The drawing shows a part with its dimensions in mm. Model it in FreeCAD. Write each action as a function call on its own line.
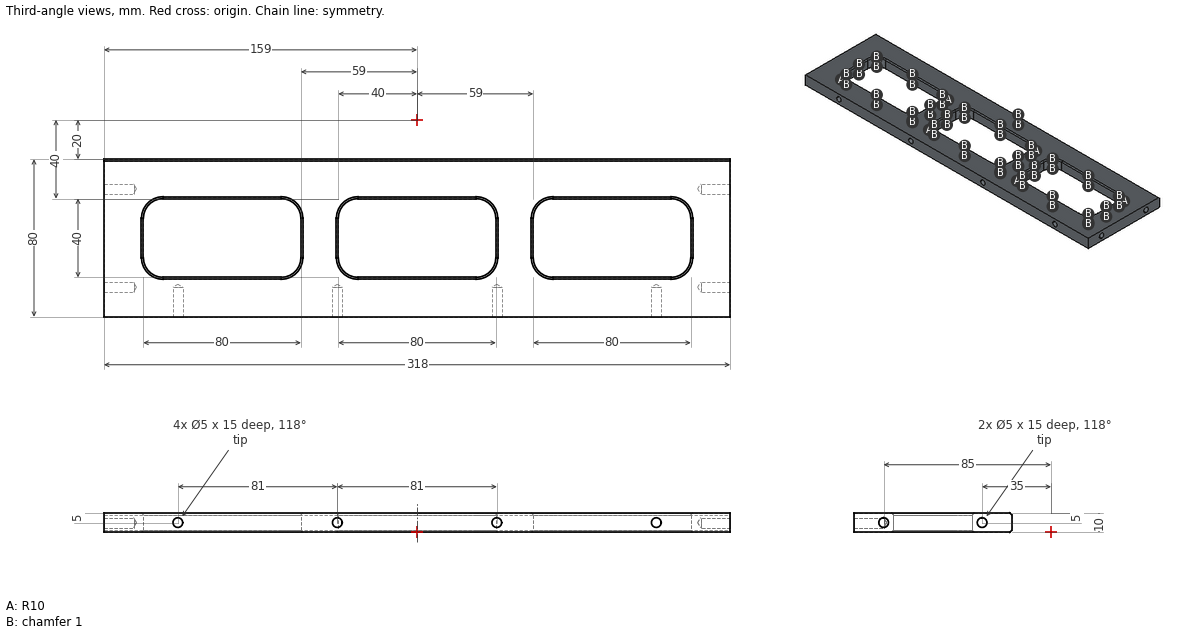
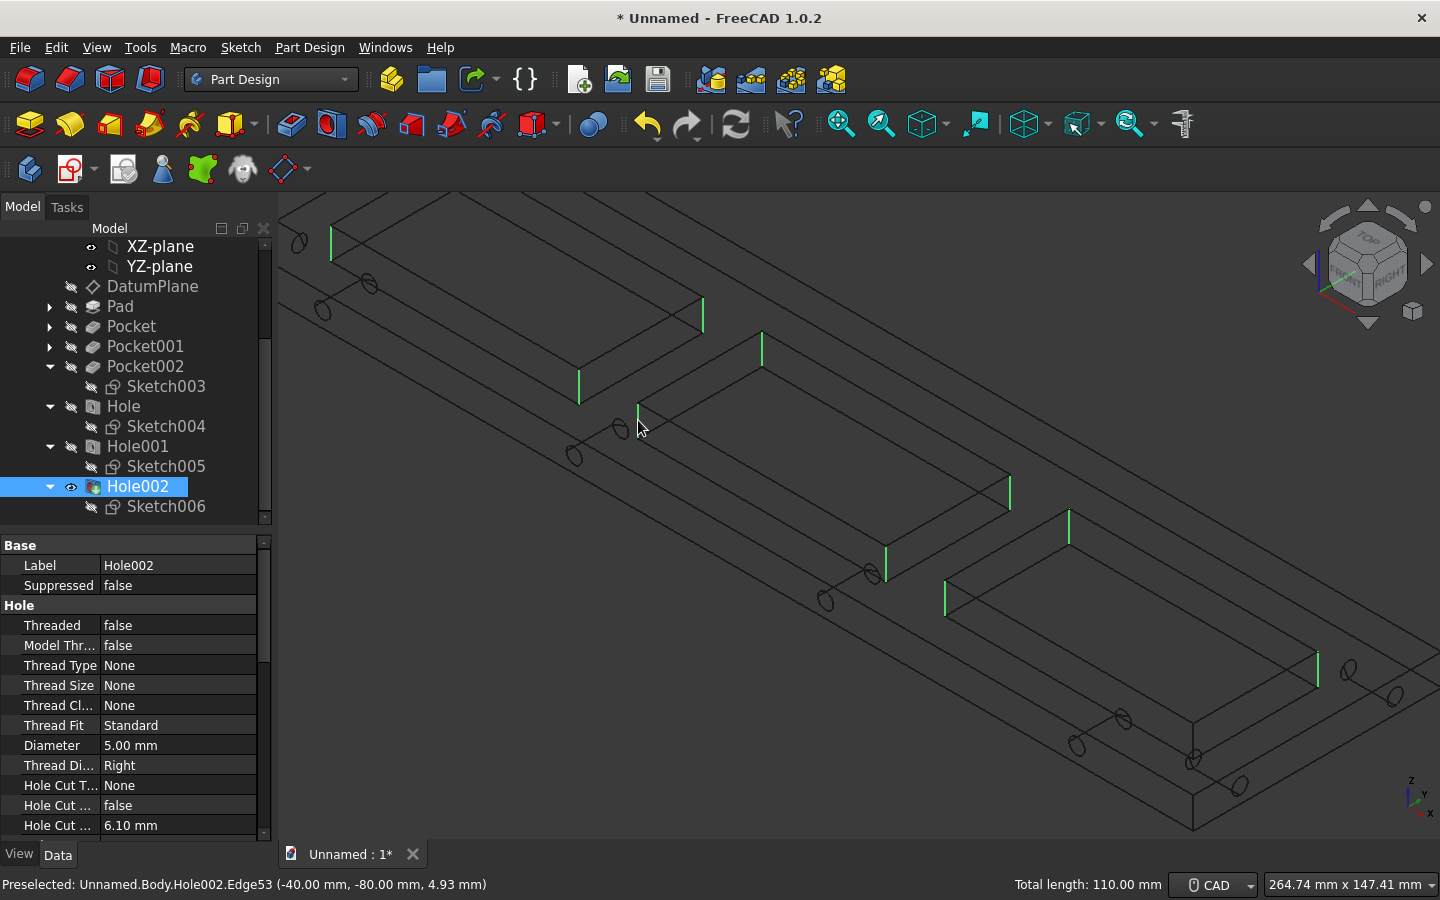
click(1193, 740, ctrl)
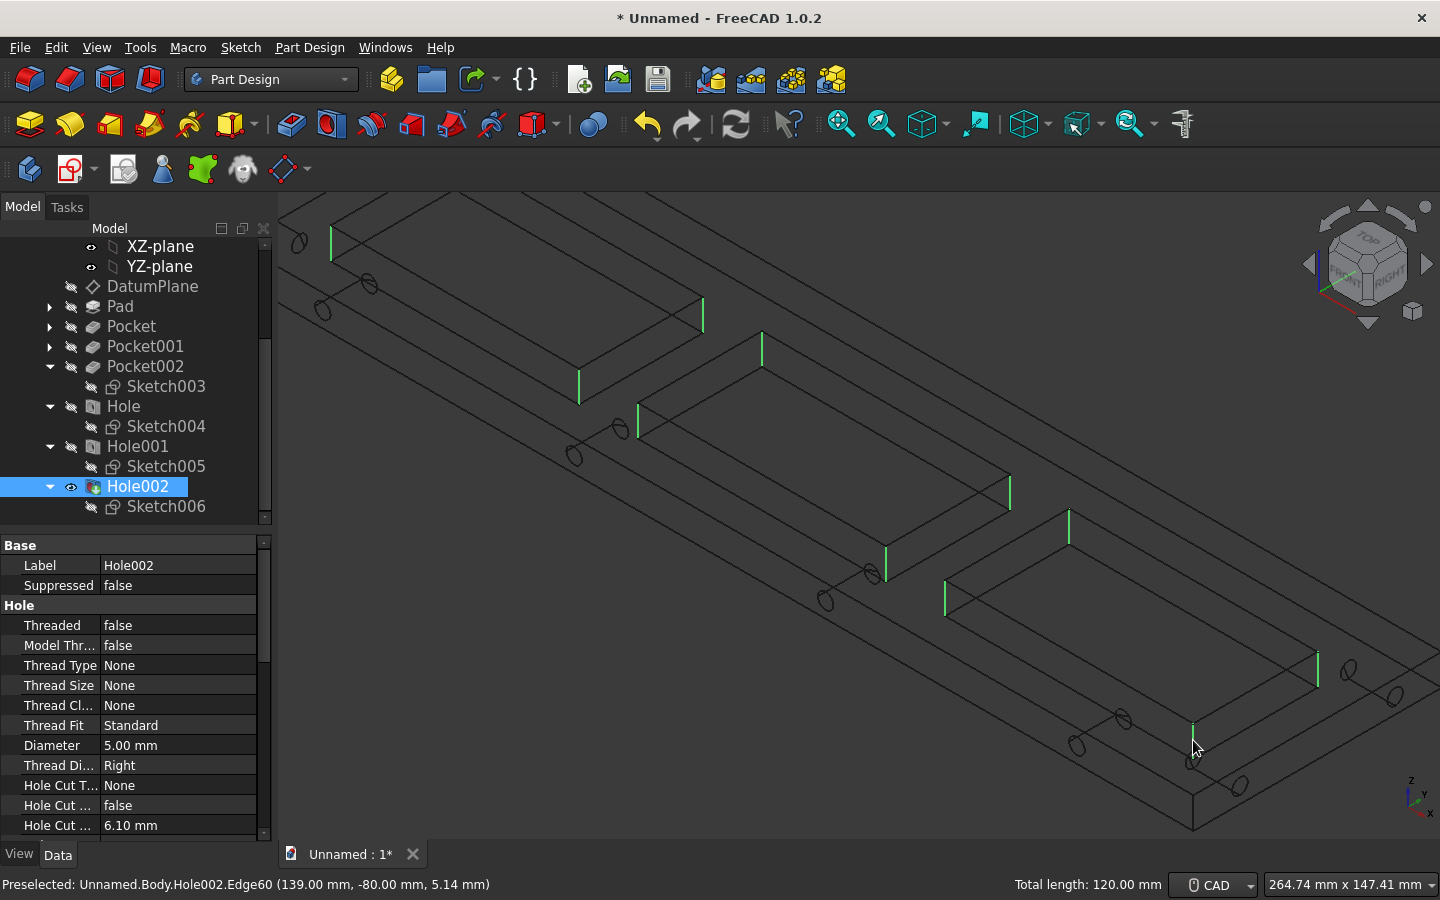
key(v)
key(1)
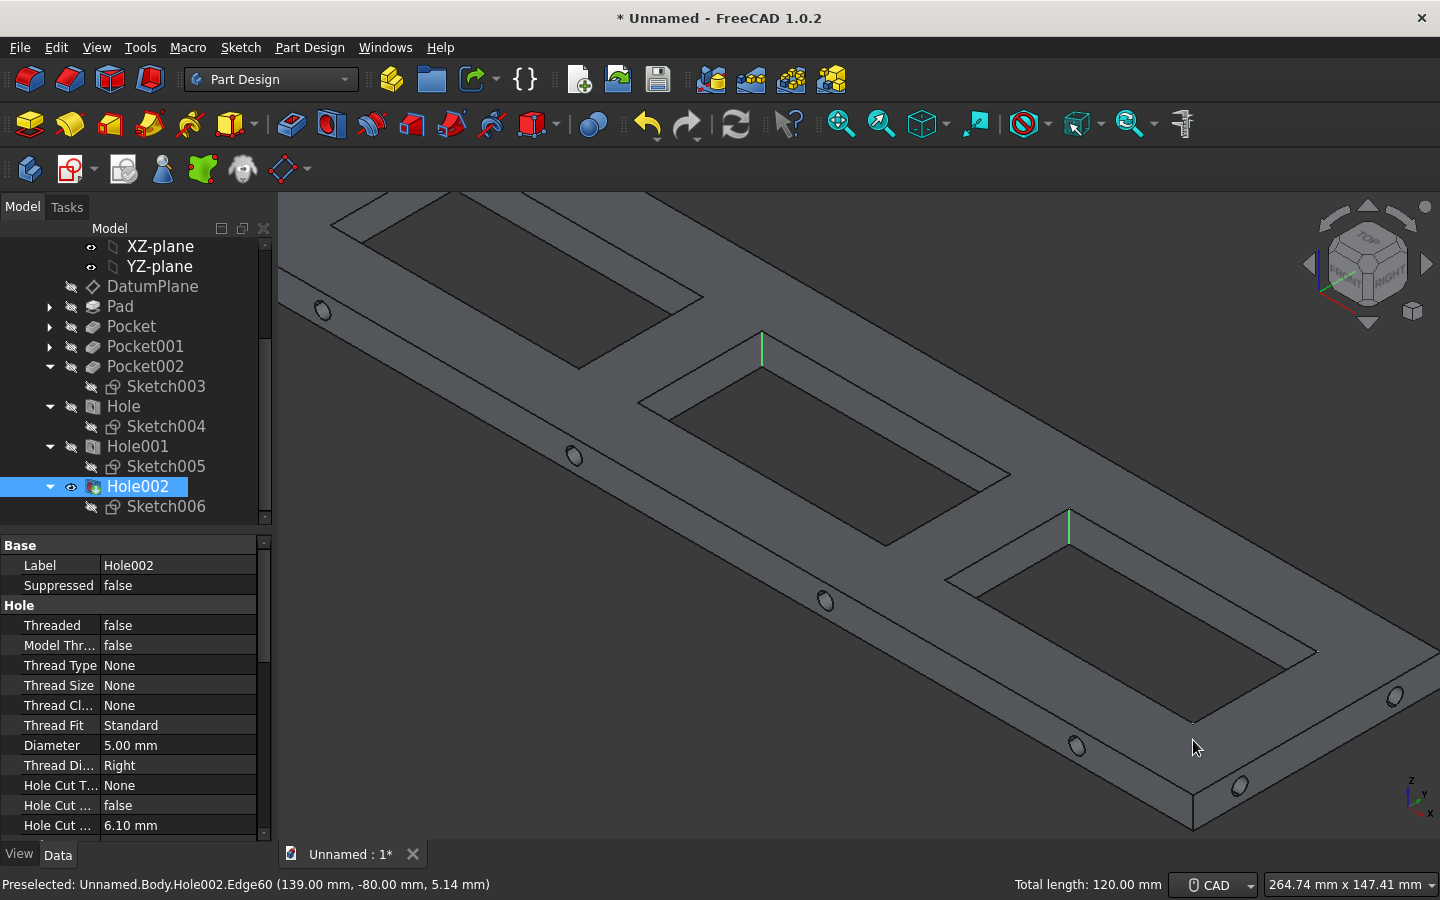
click(30, 80)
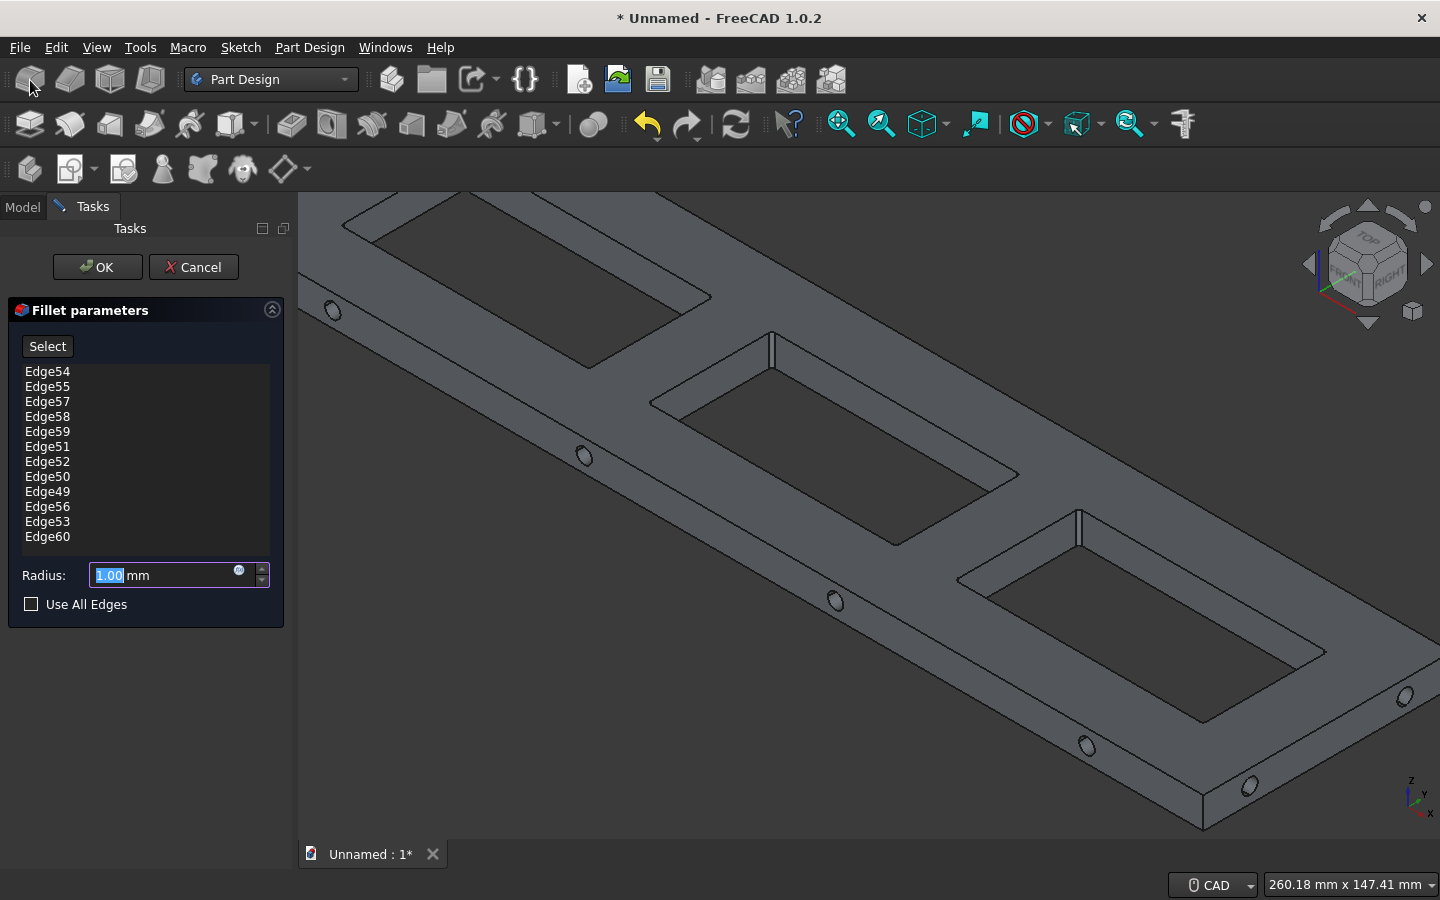
text(10)
key(Tab)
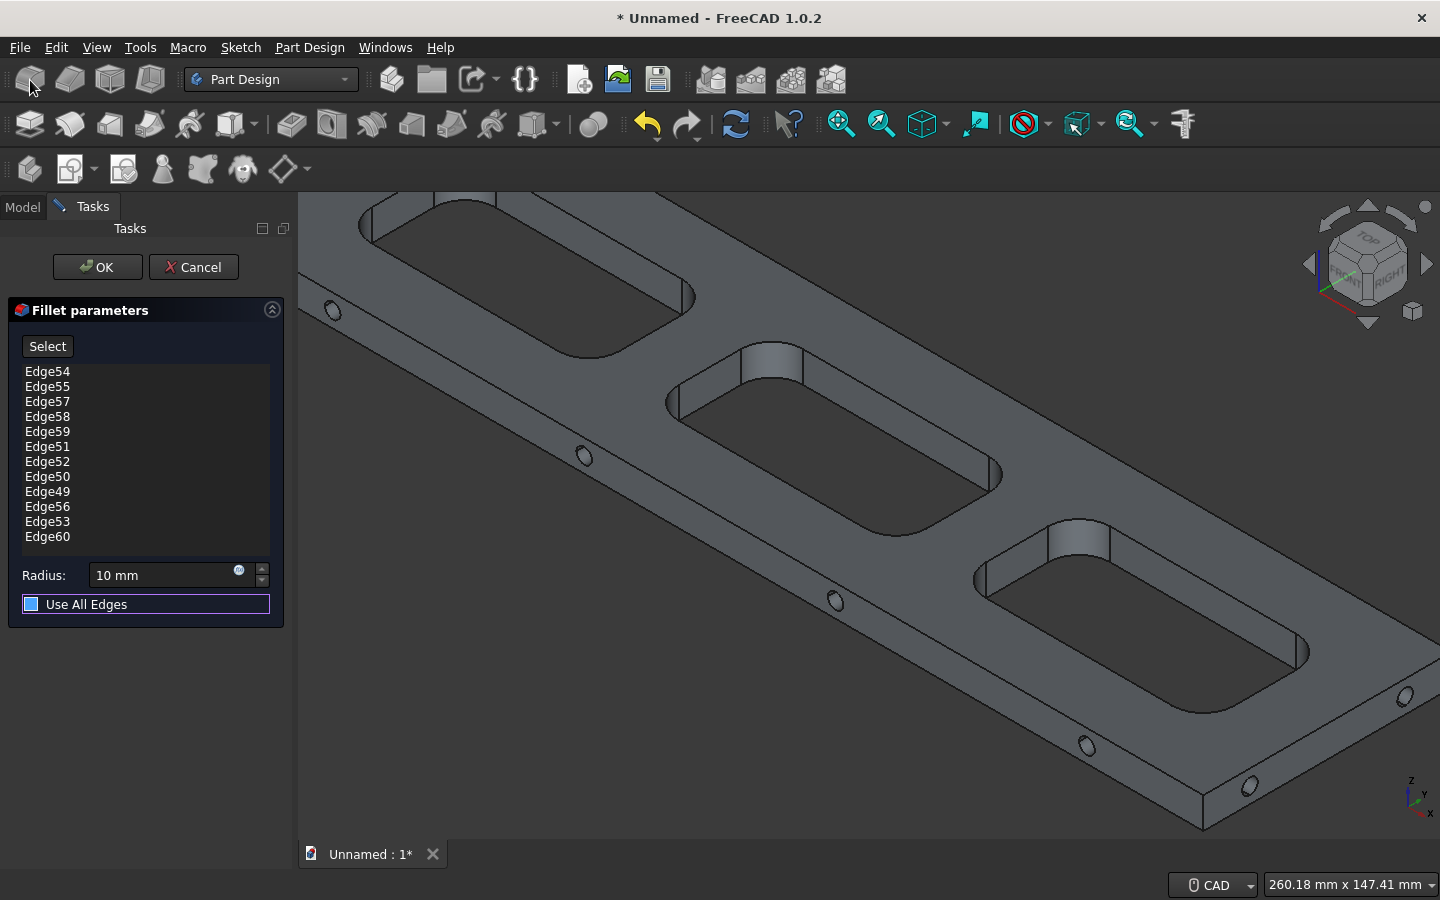
click(98, 267)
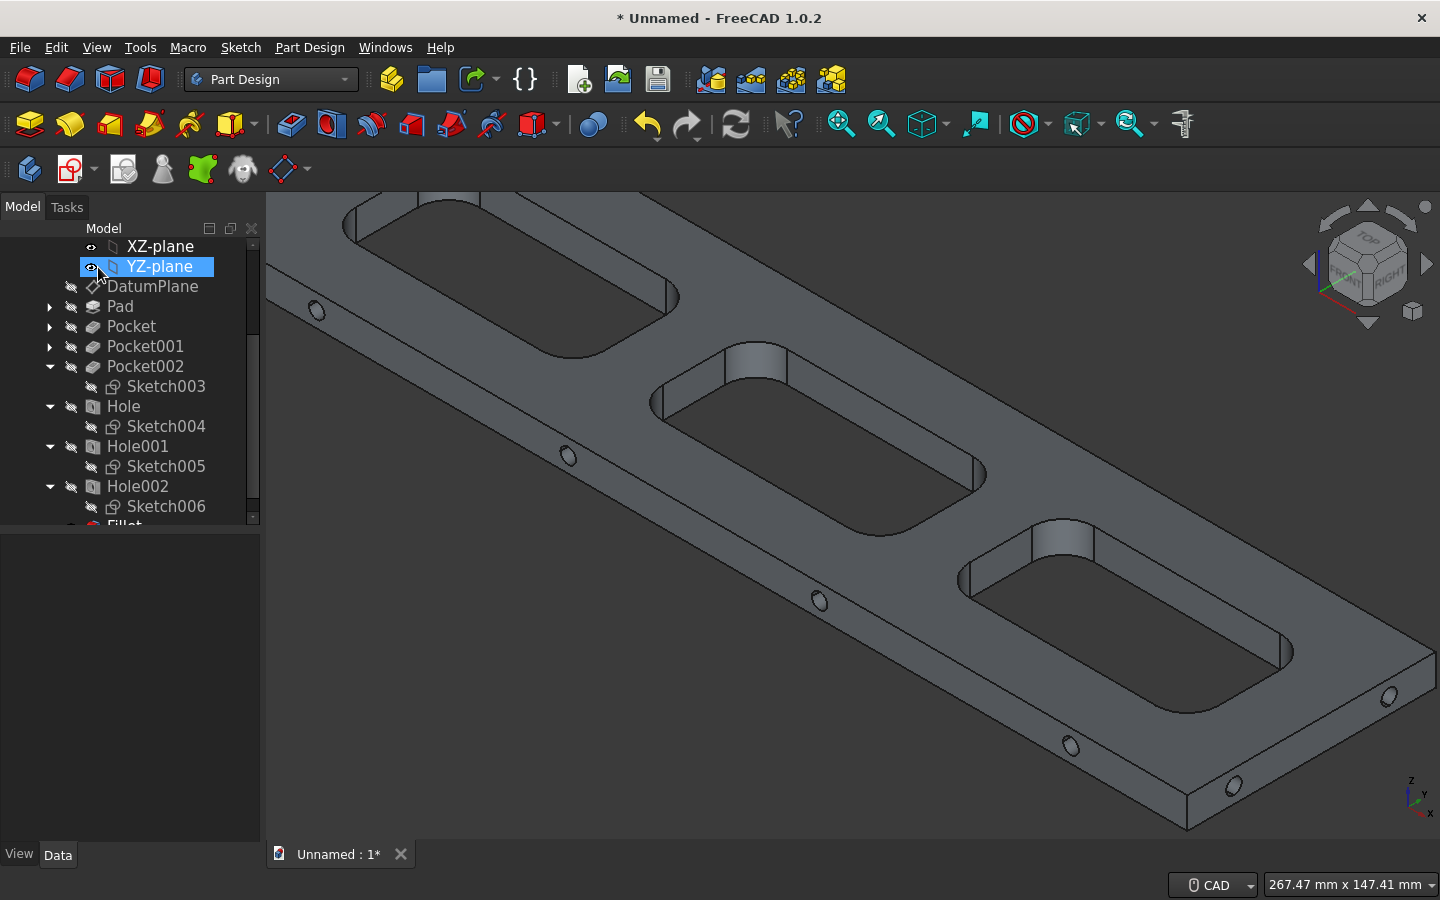
click(842, 124)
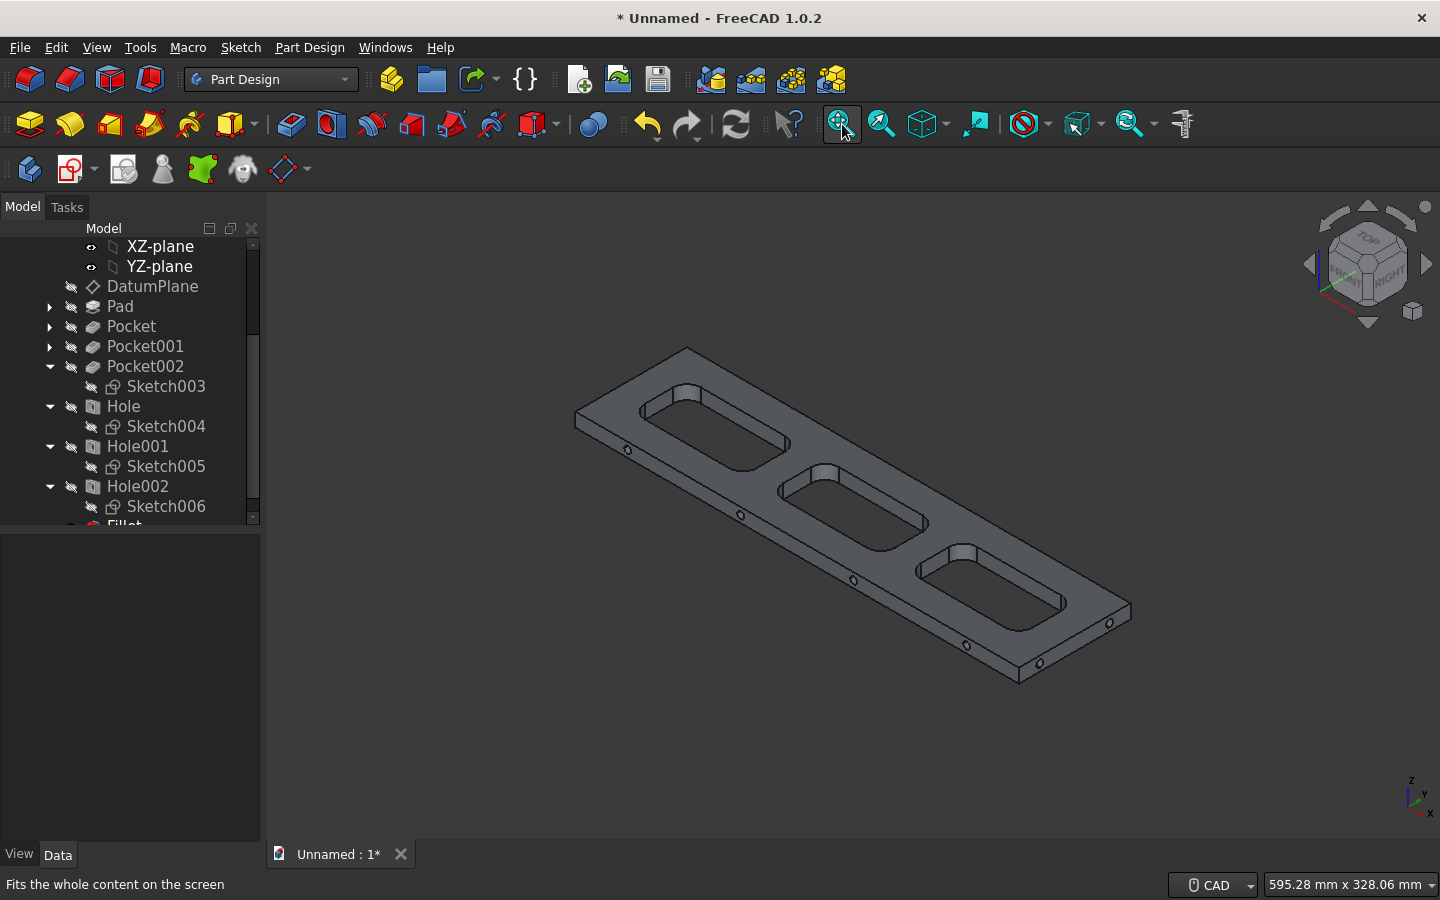
click(881, 490)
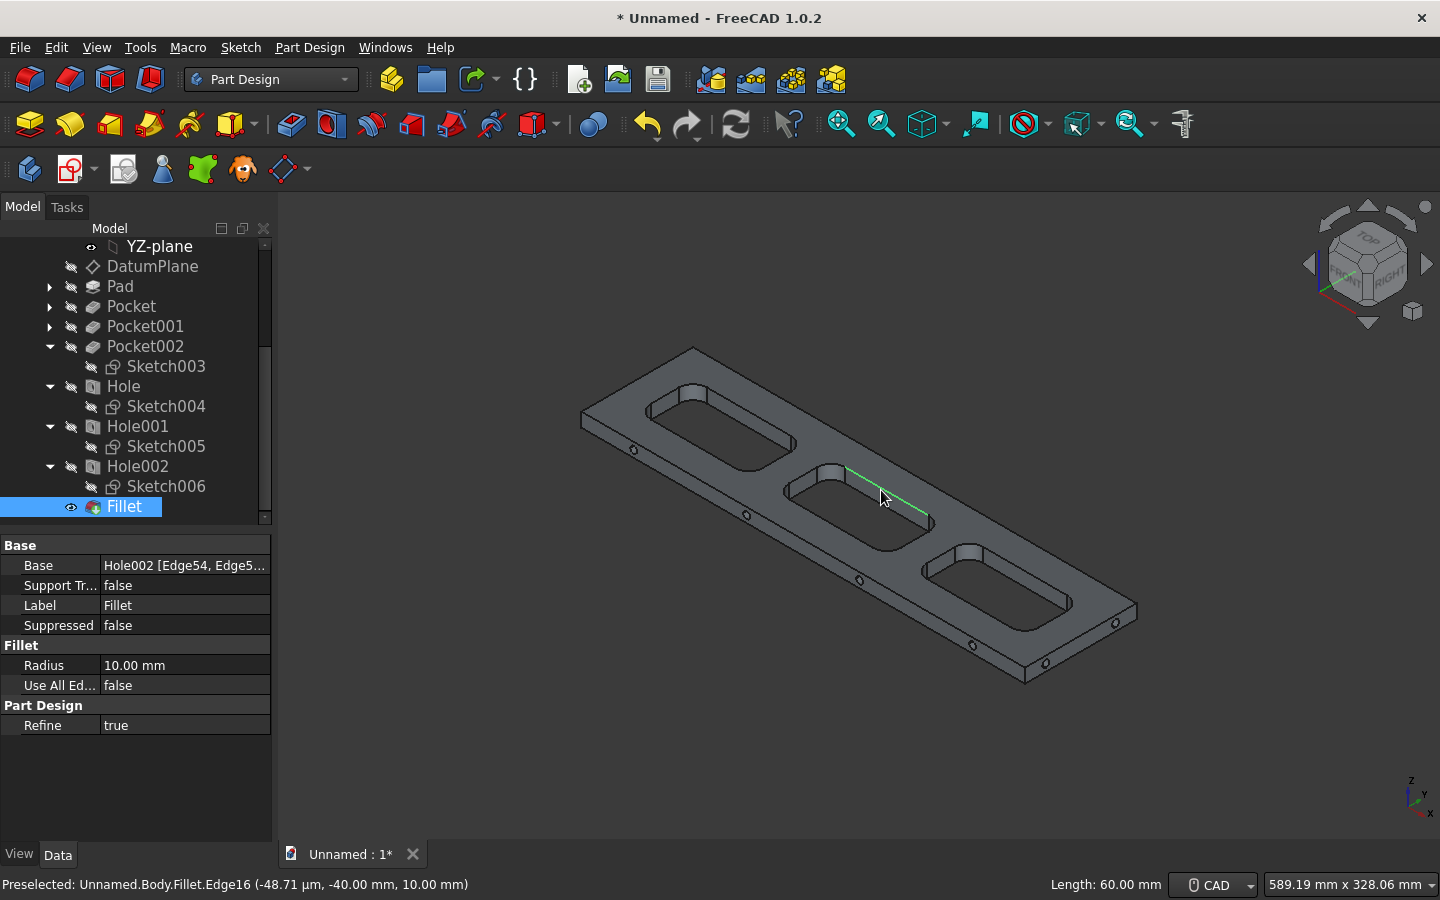
click(1025, 570, ctrl)